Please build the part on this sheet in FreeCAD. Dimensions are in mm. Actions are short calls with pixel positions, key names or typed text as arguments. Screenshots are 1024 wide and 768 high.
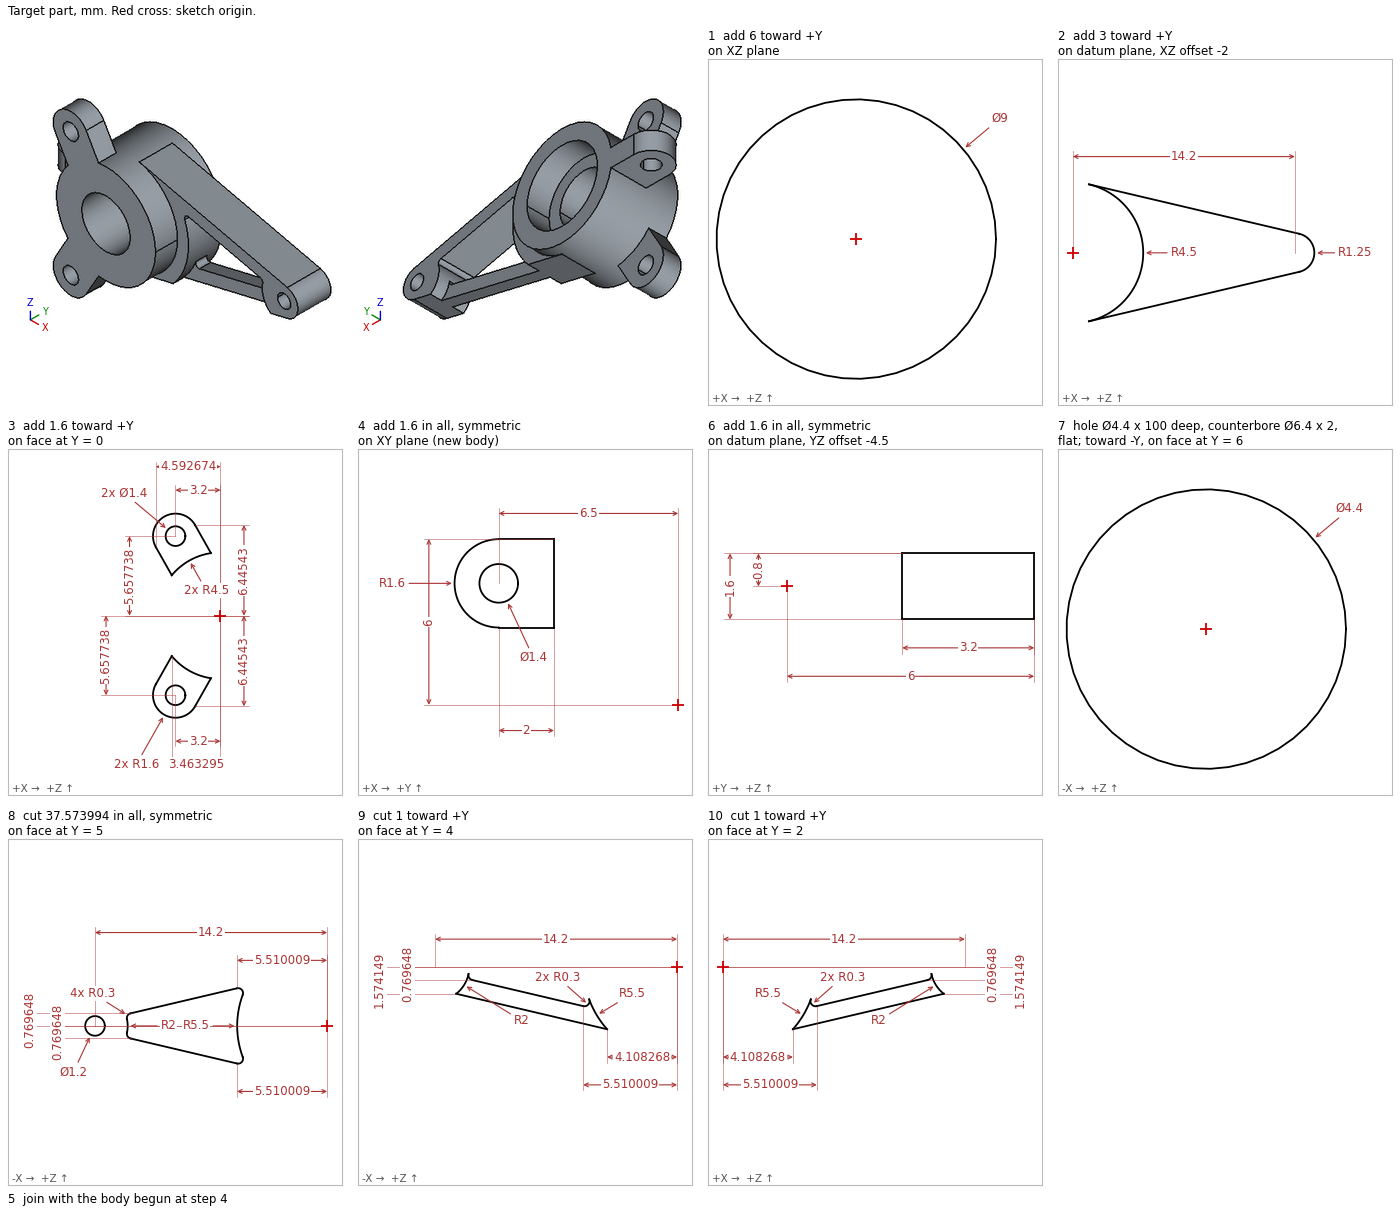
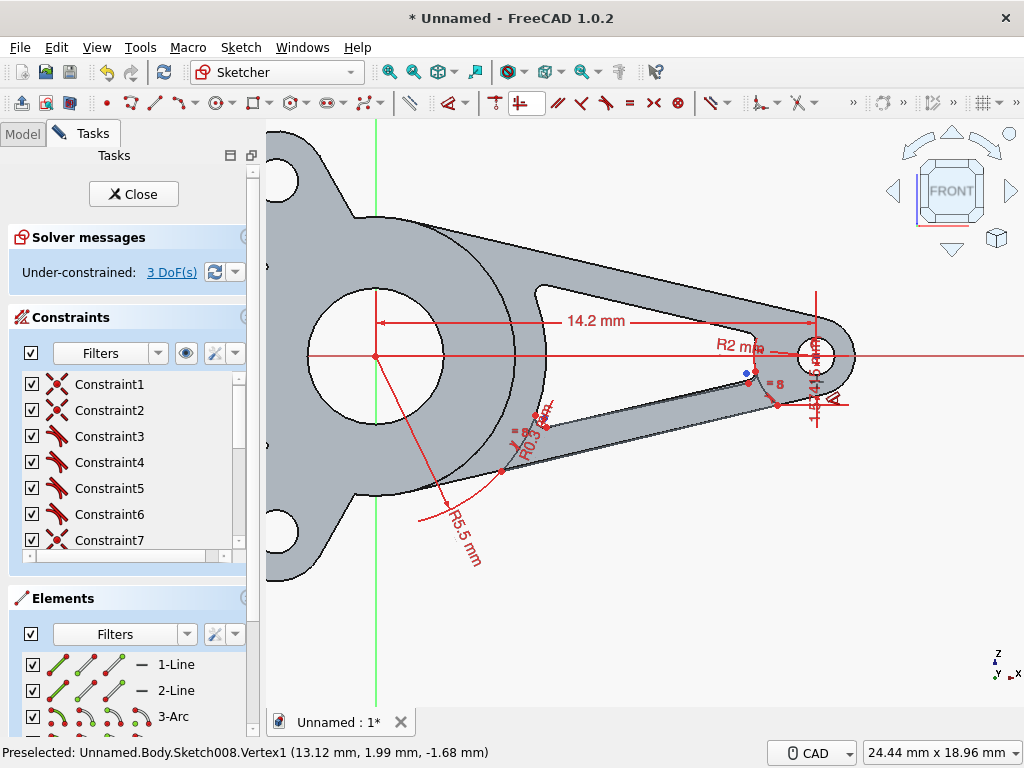
click(501, 472)
click(439, 506)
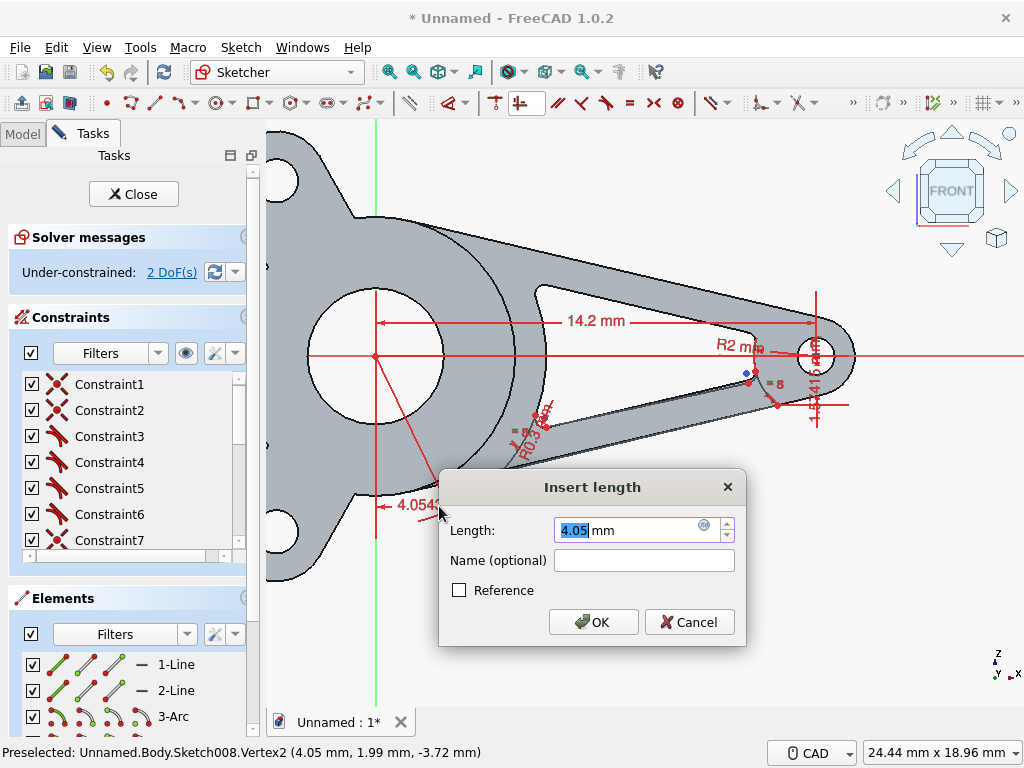
text(4.108268)
key(Return)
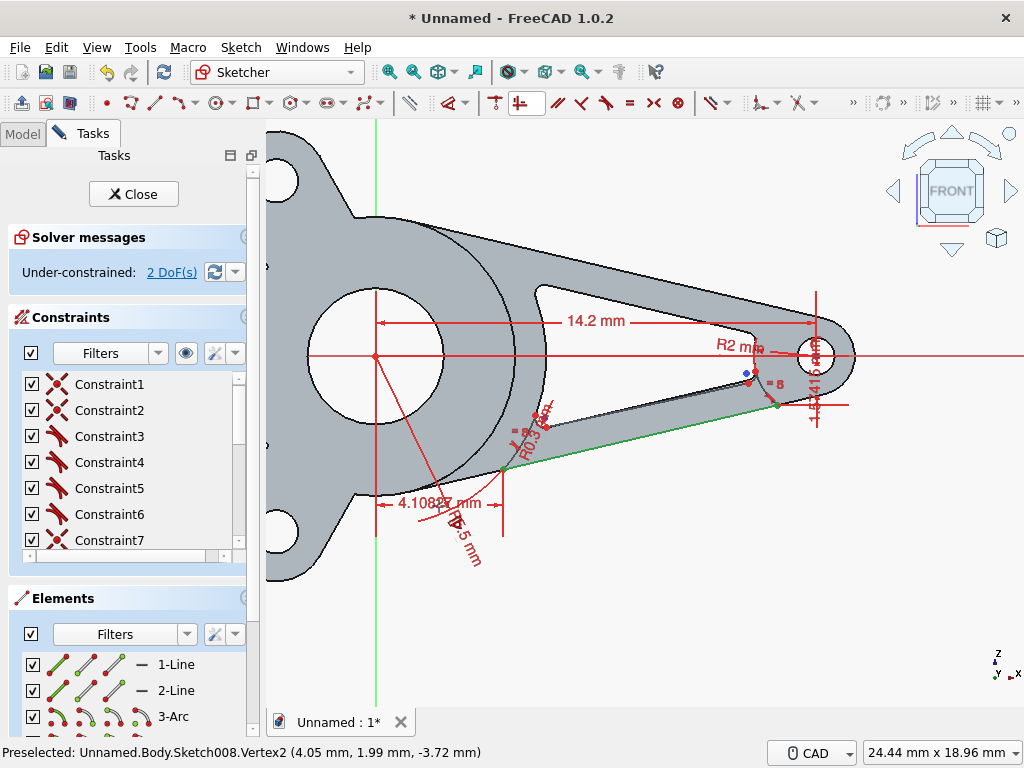
scroll(547, 427, up, 2)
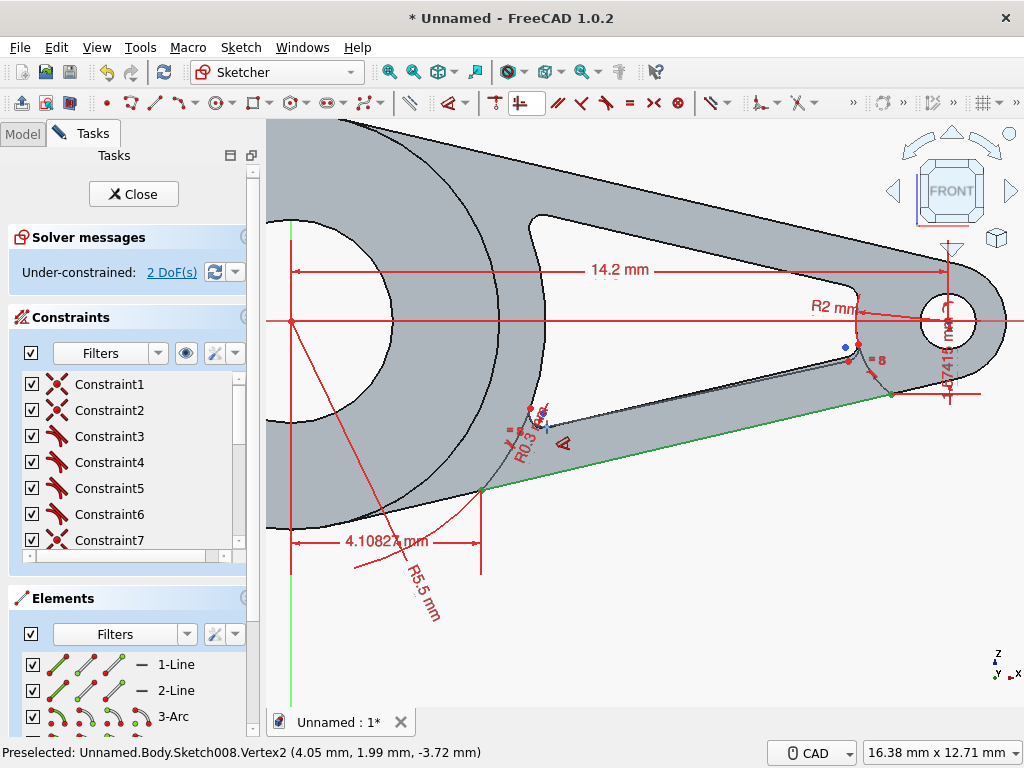
click(546, 427)
click(420, 287)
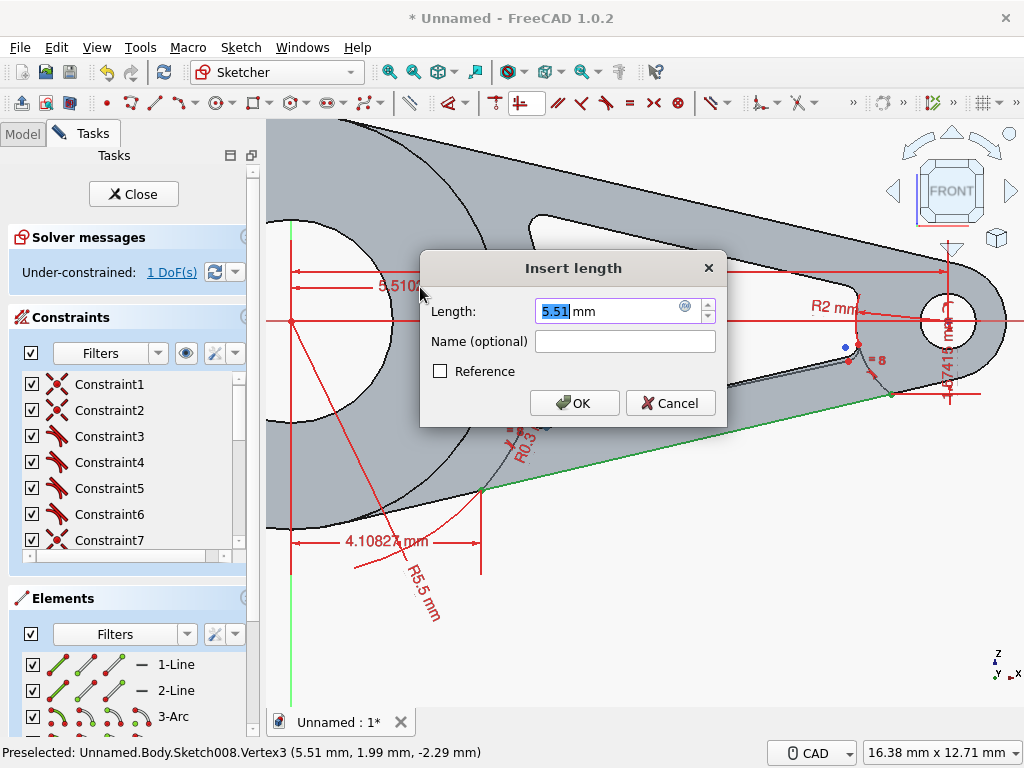
text(5.510009)
key(Return)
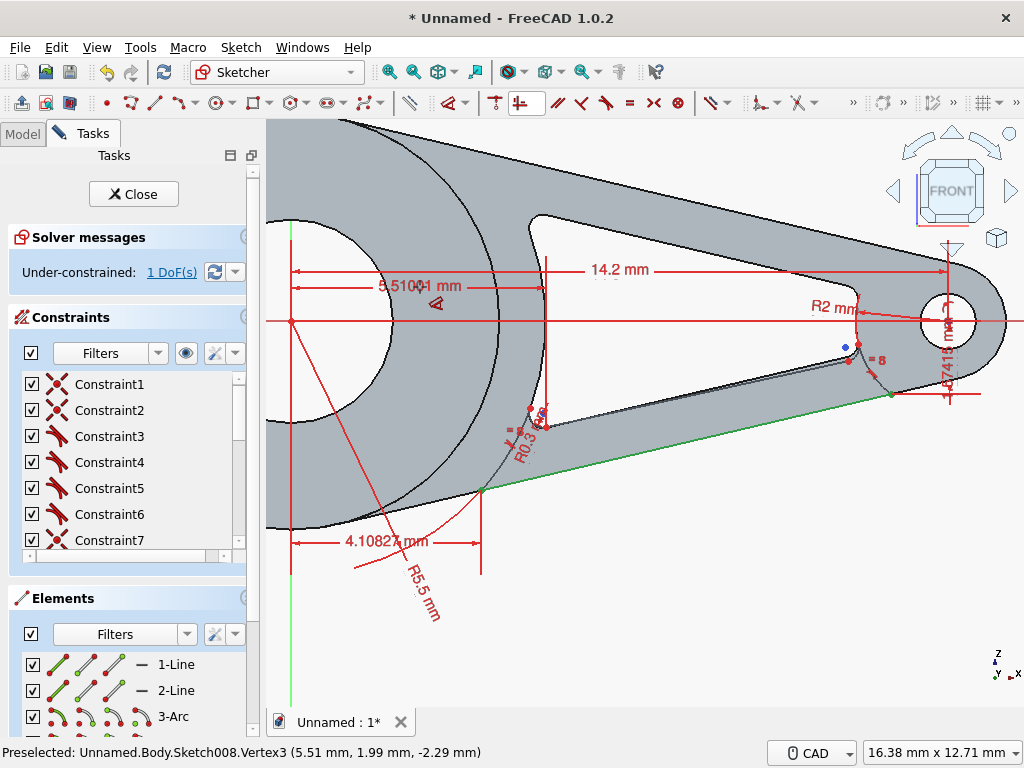
click(848, 361)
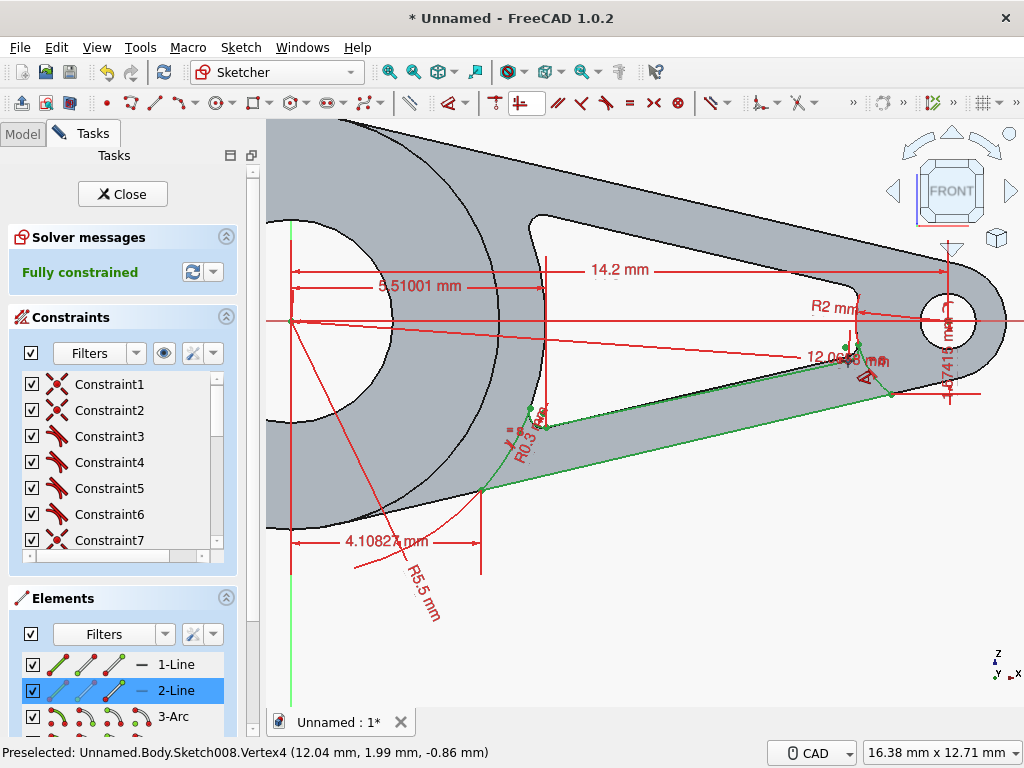
key(Escape)
key(Escape)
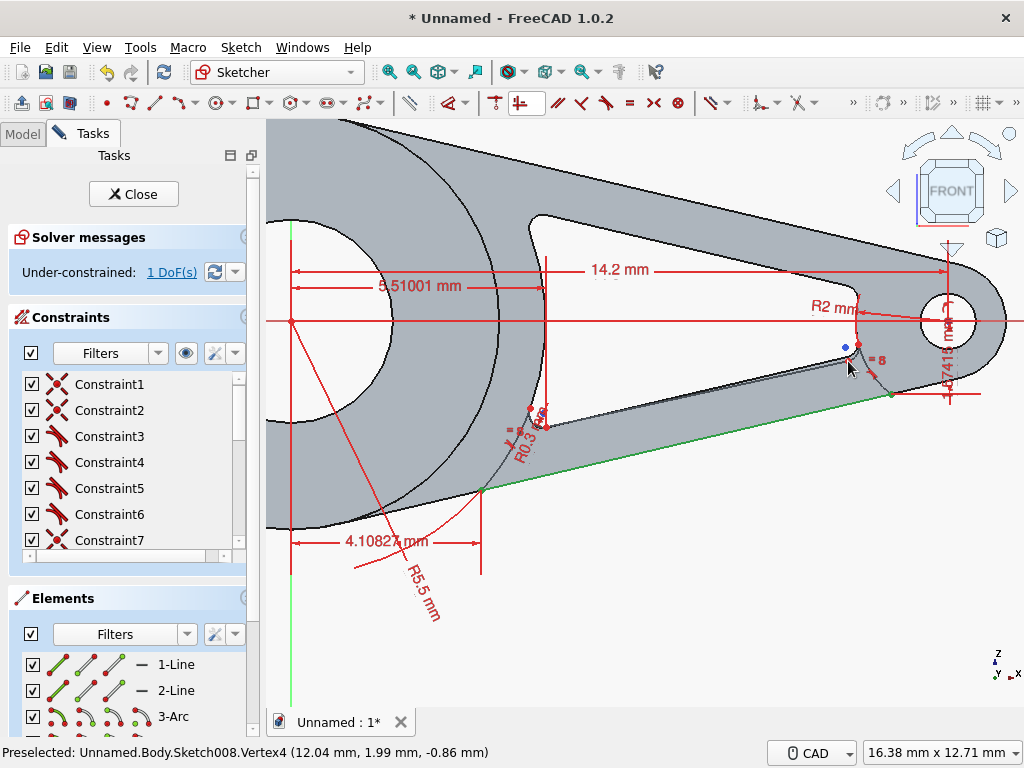
click(848, 361)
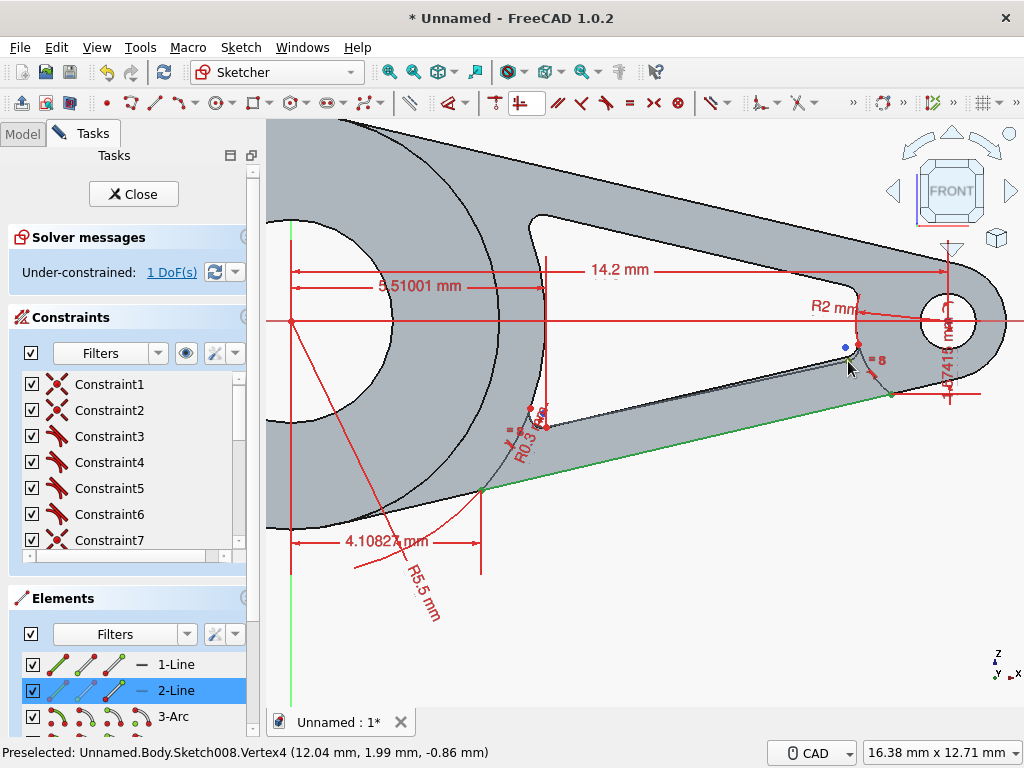
key(i)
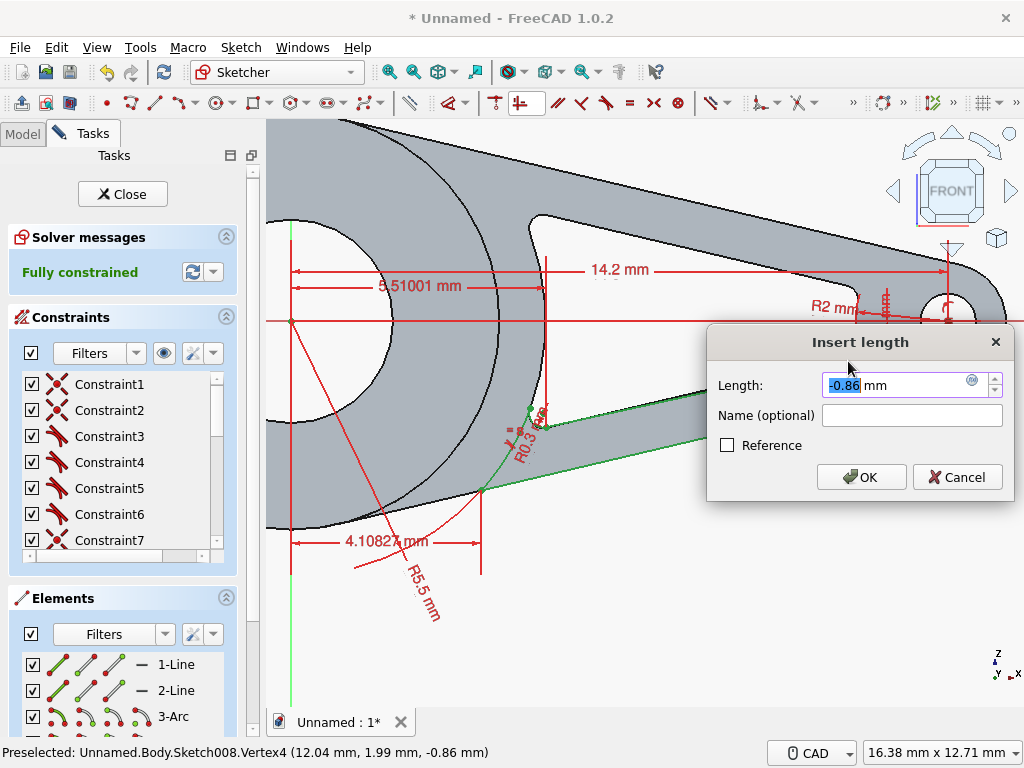
text(-0.769648)
key(Return)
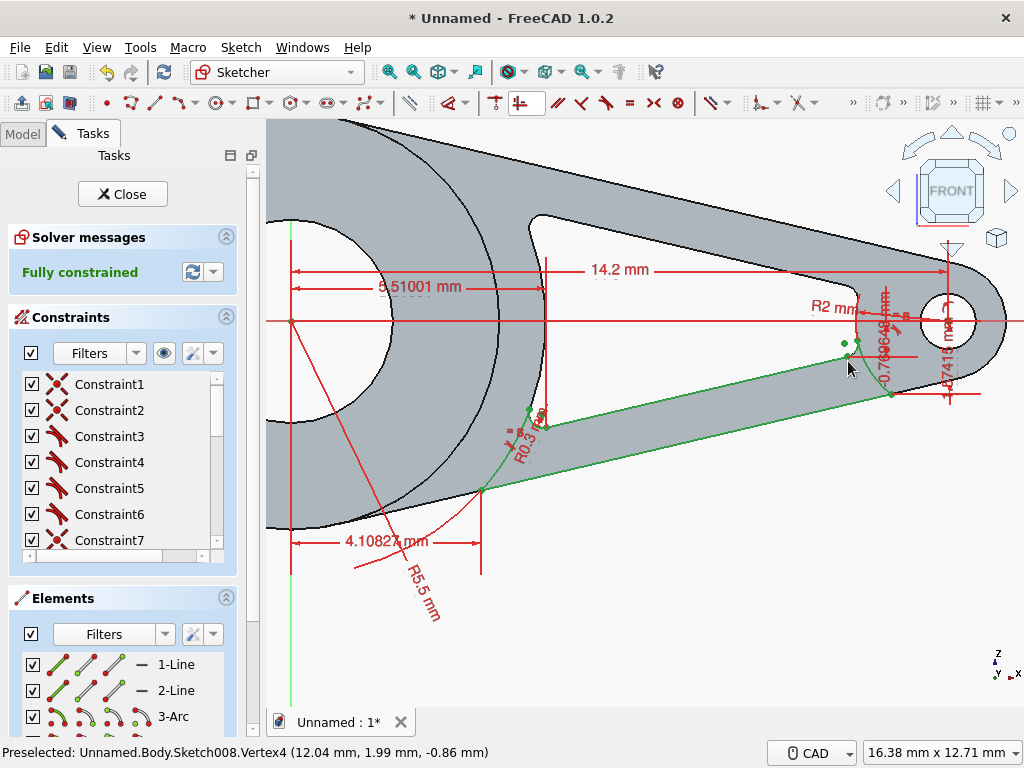
click(123, 194)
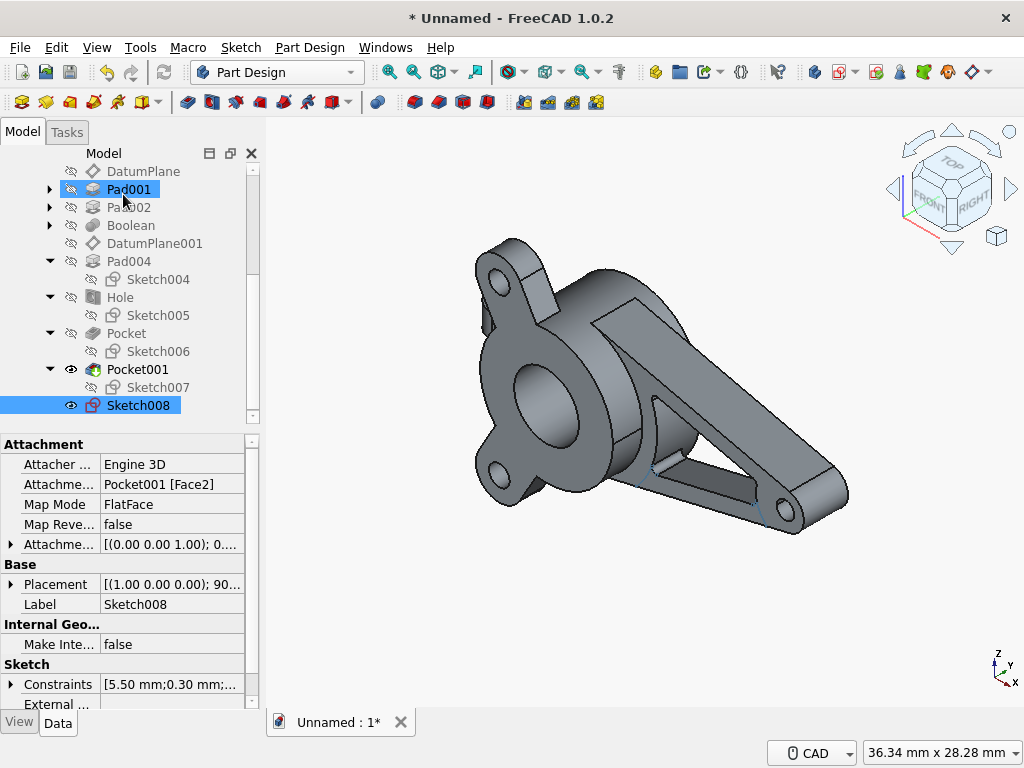
click(188, 102)